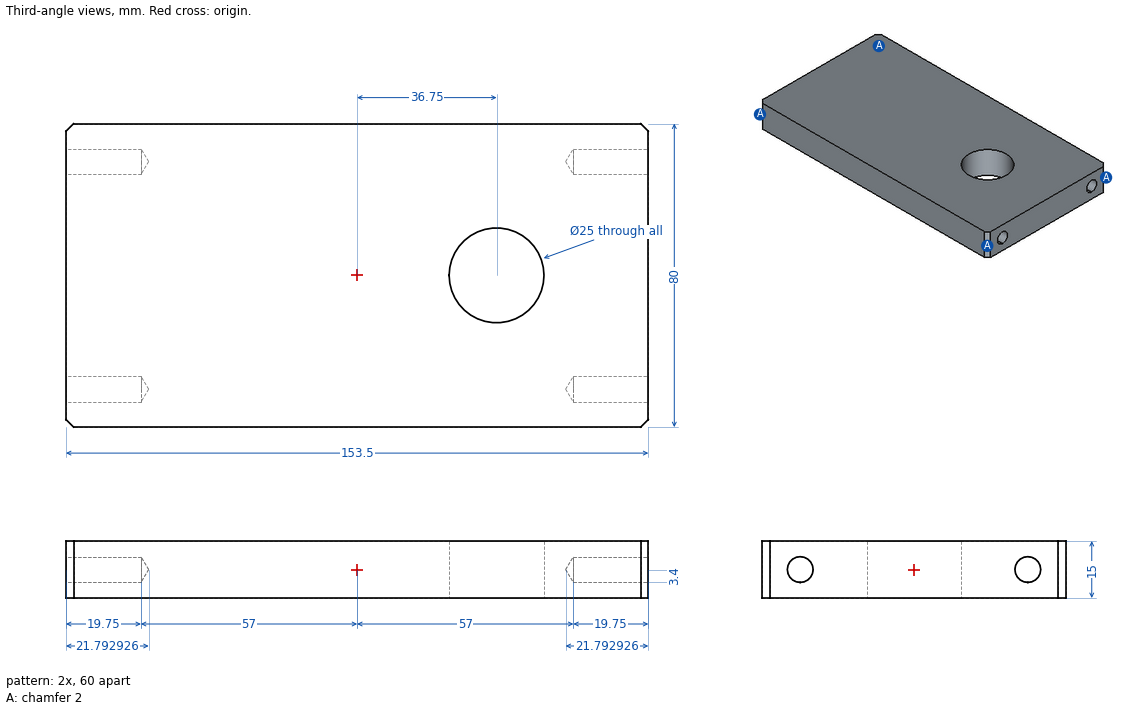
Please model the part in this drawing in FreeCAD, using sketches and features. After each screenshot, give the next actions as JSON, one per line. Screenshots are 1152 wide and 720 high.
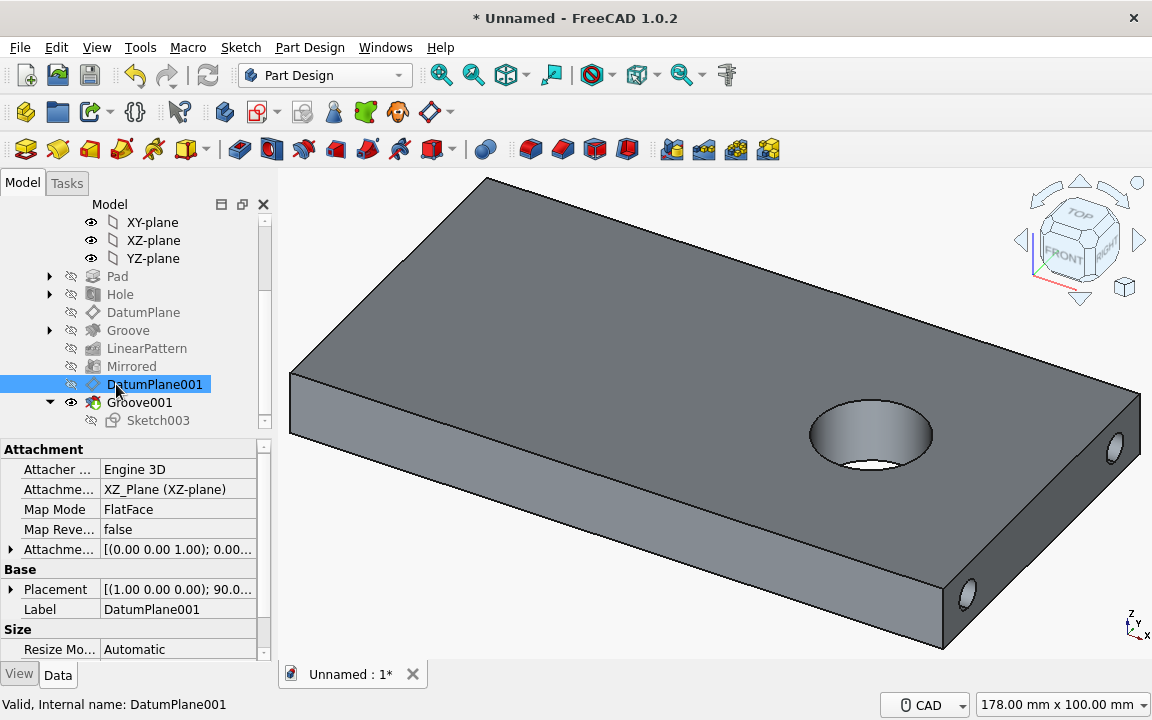
{"action": "left_click", "coordinate": [943, 618]}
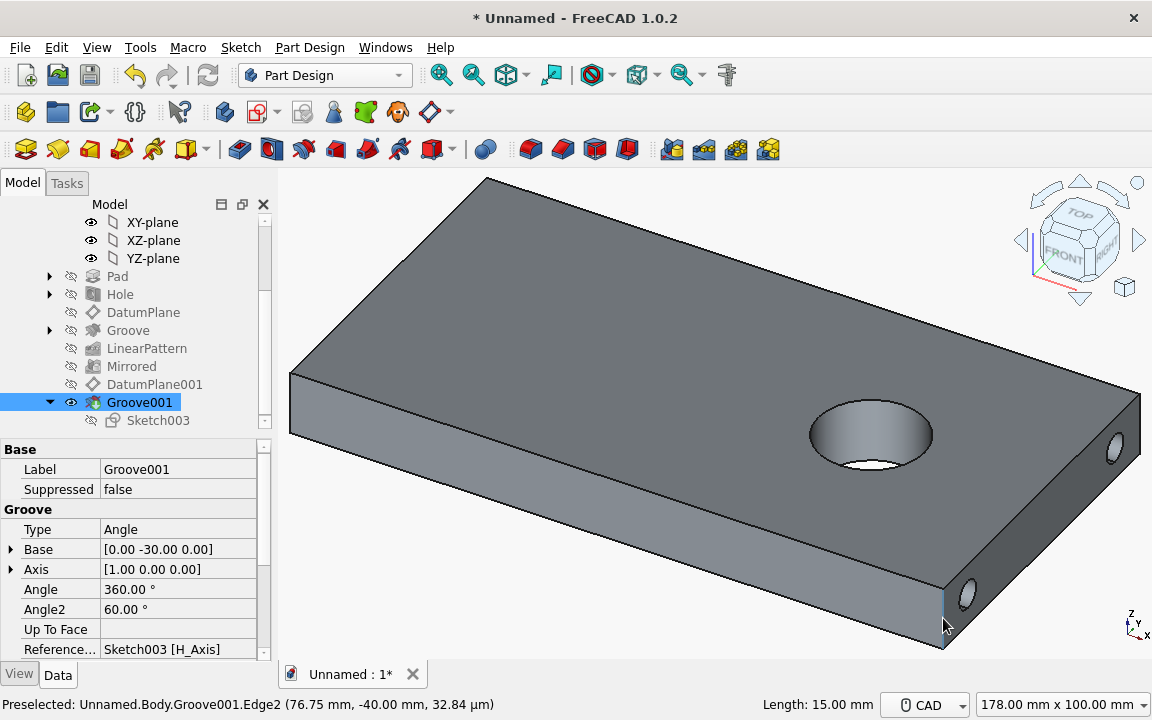
{"action": "key", "text": "0"}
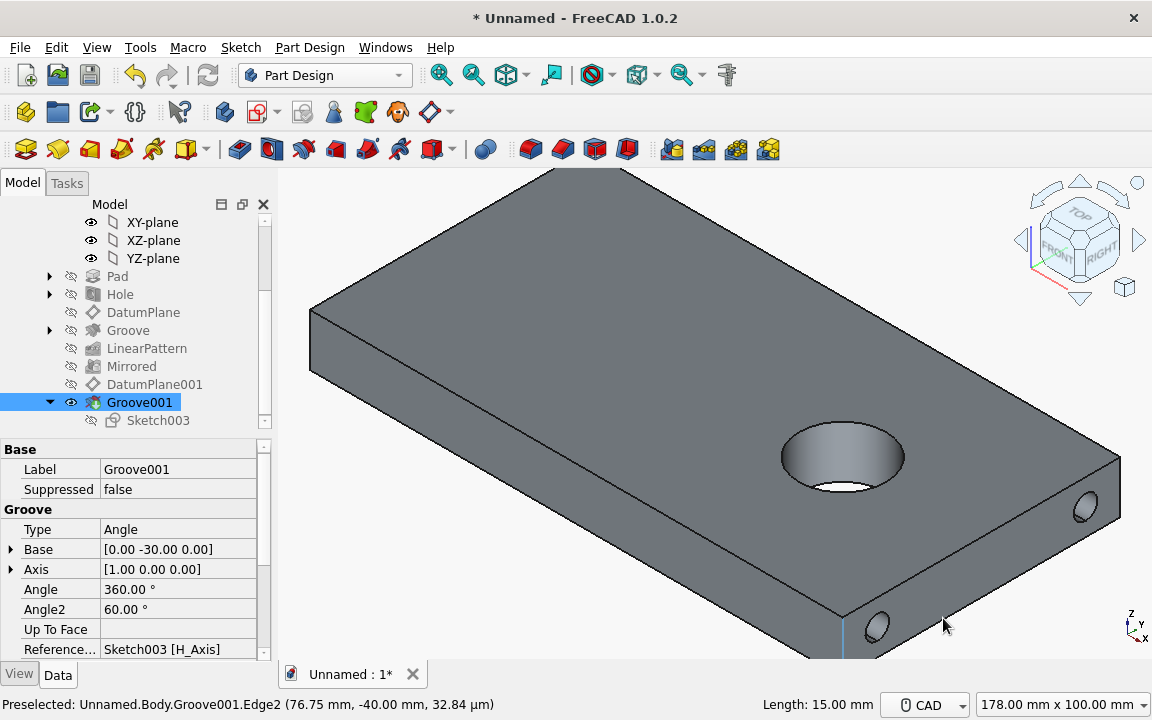
{"action": "left_click", "coordinate": [442, 76]}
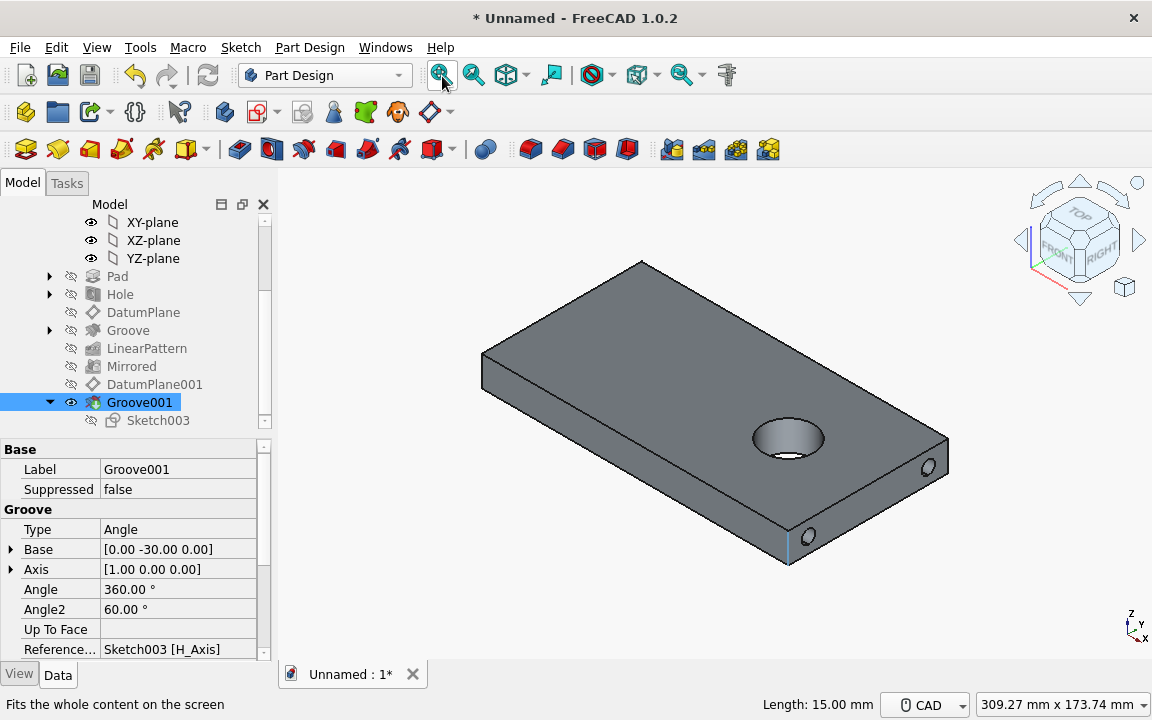
{"action": "key", "text": "2"}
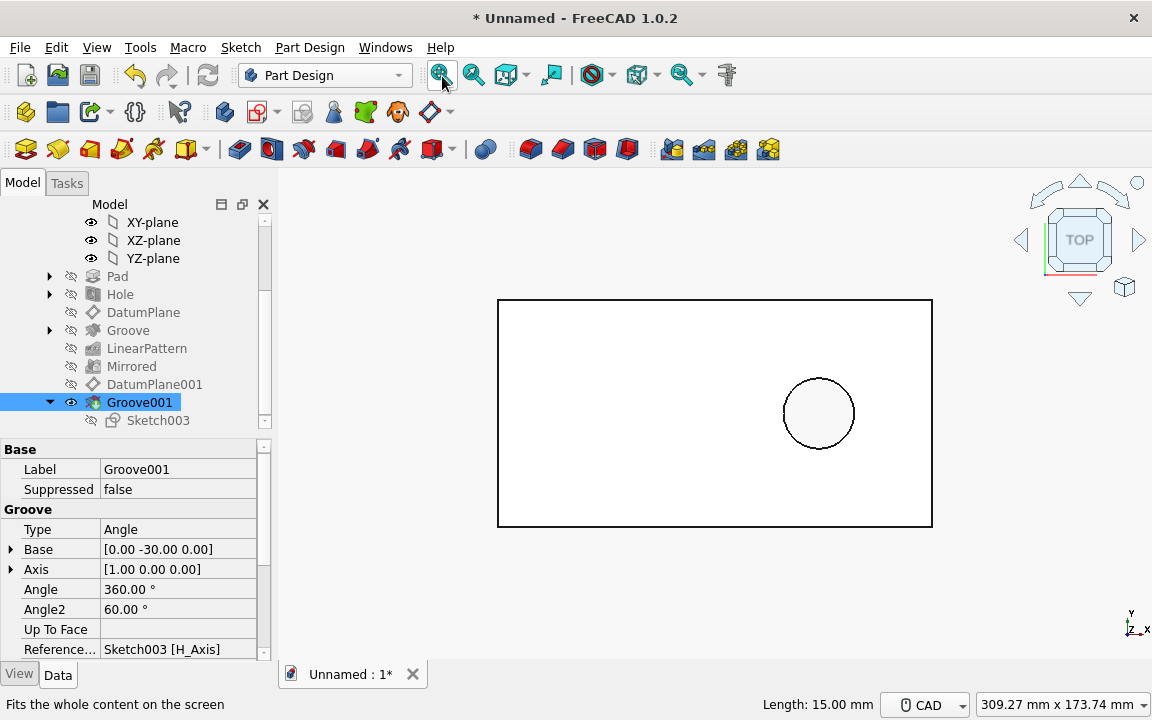
{"action": "key", "text": "1"}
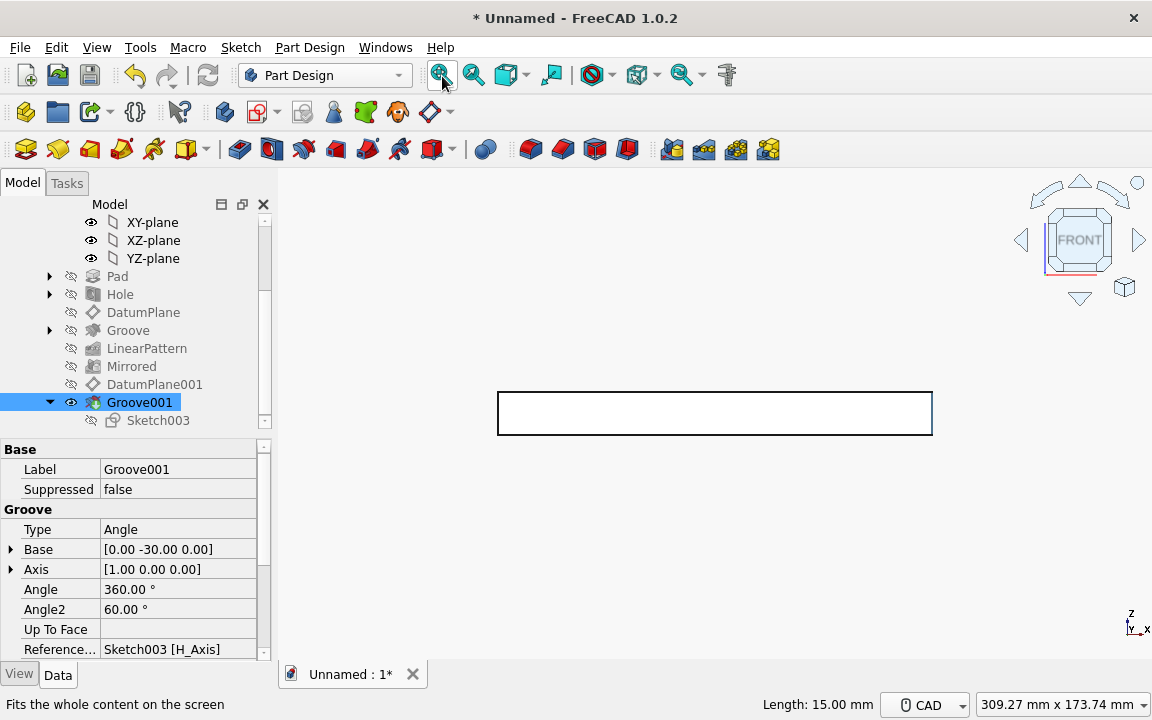
{"action": "left_click", "coordinate": [498, 413], "text": "ctrl"}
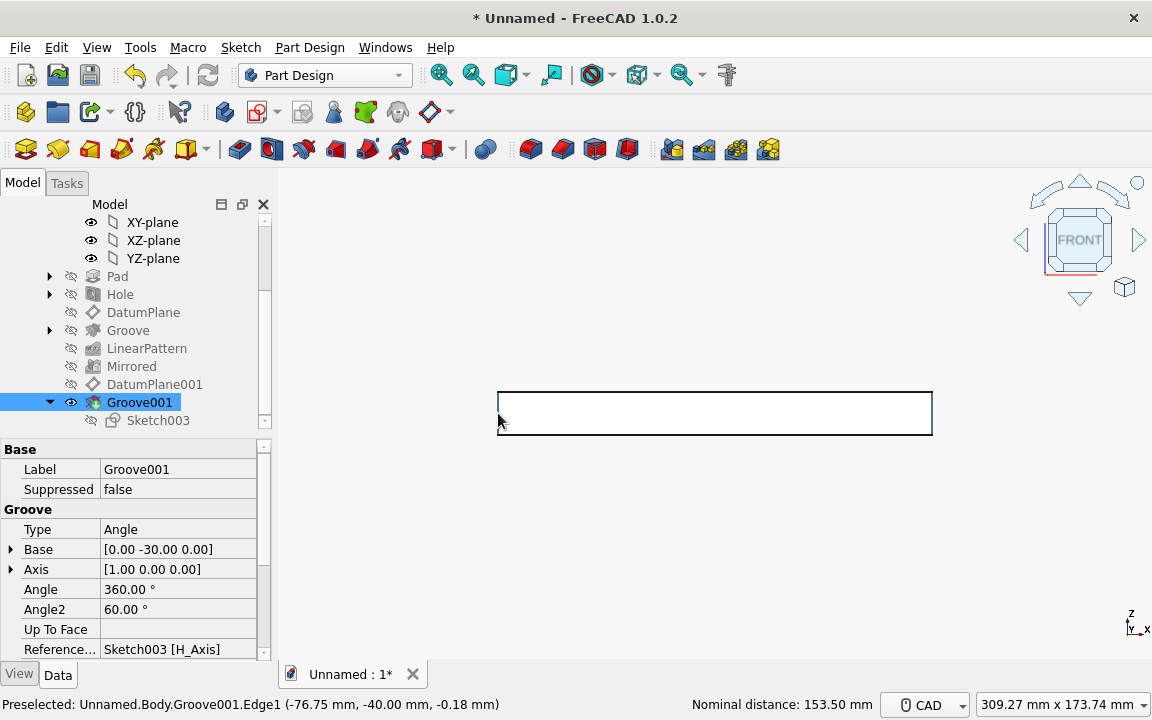
{"action": "key", "text": "3"}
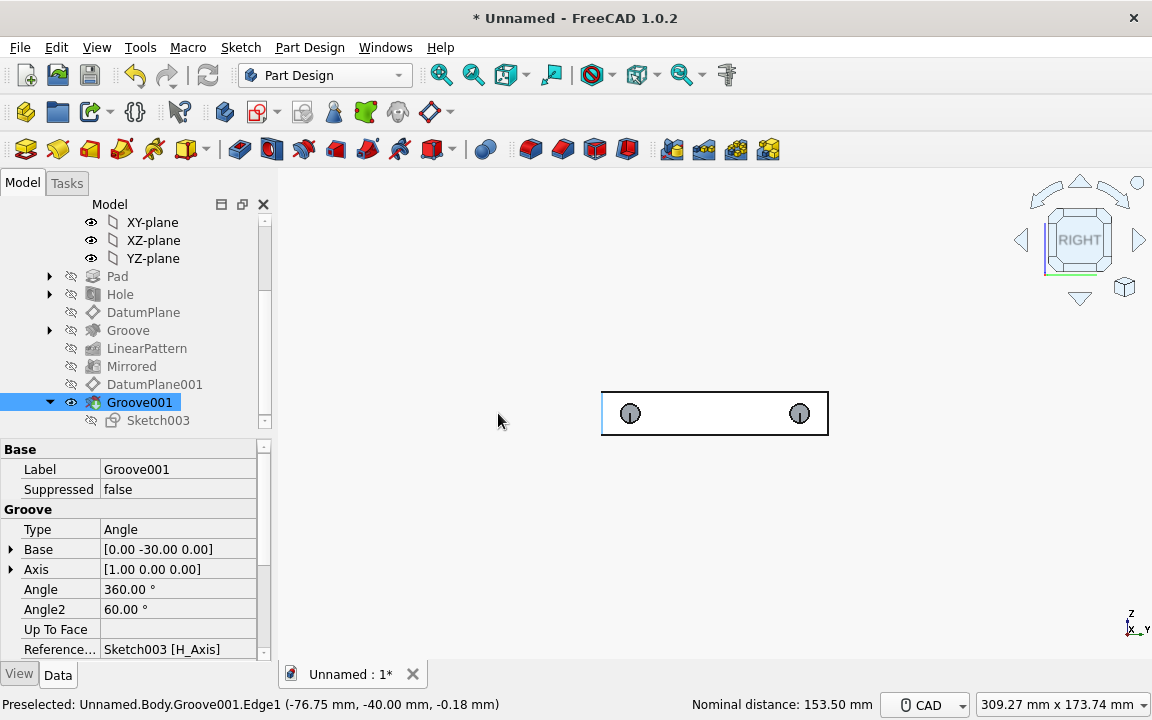
{"action": "key", "text": "v f"}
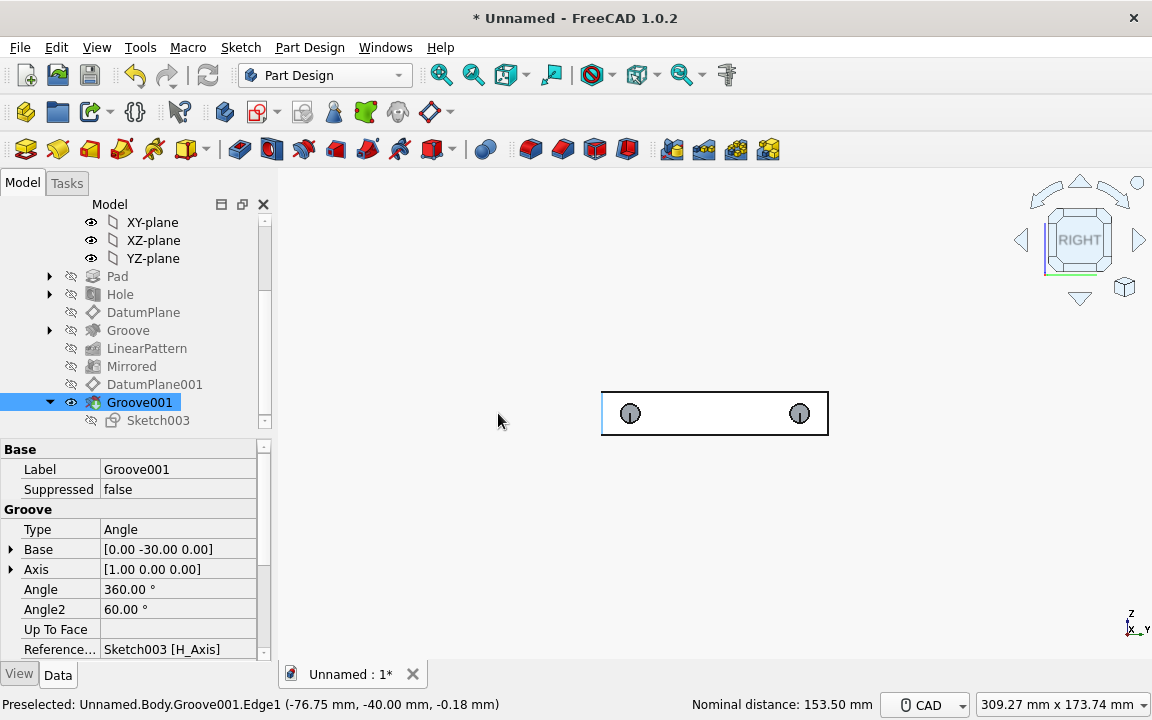
{"action": "left_click", "coordinate": [828, 412], "text": "ctrl"}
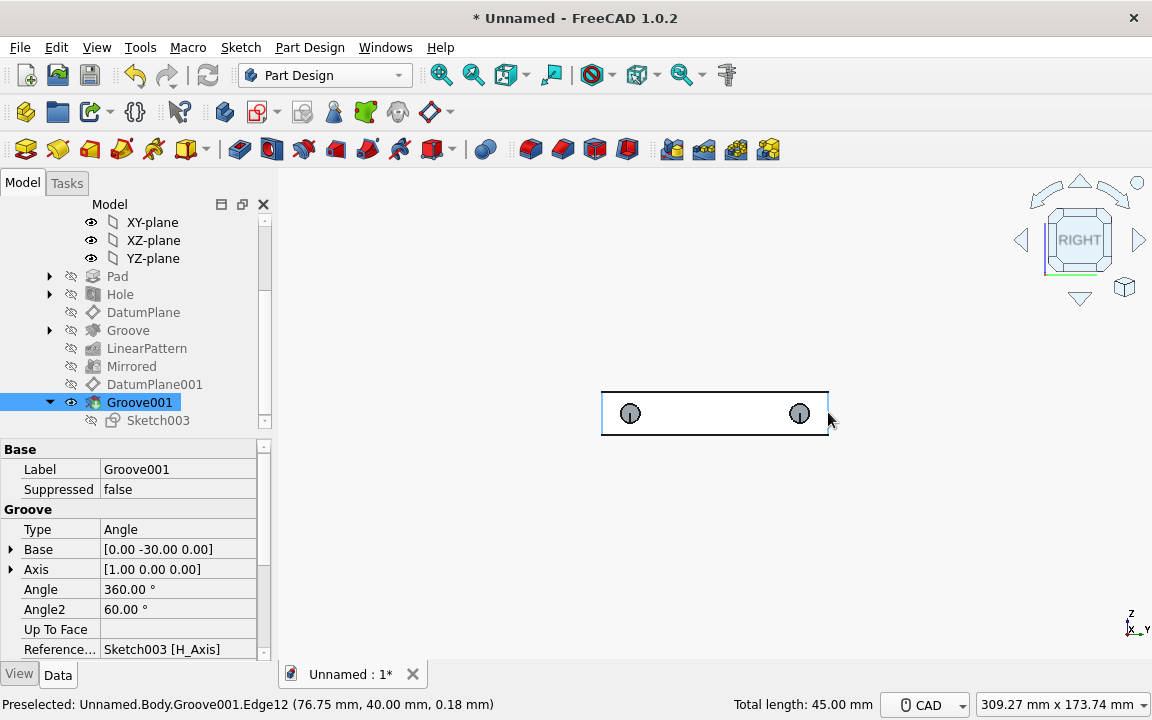
{"action": "key", "text": "5"}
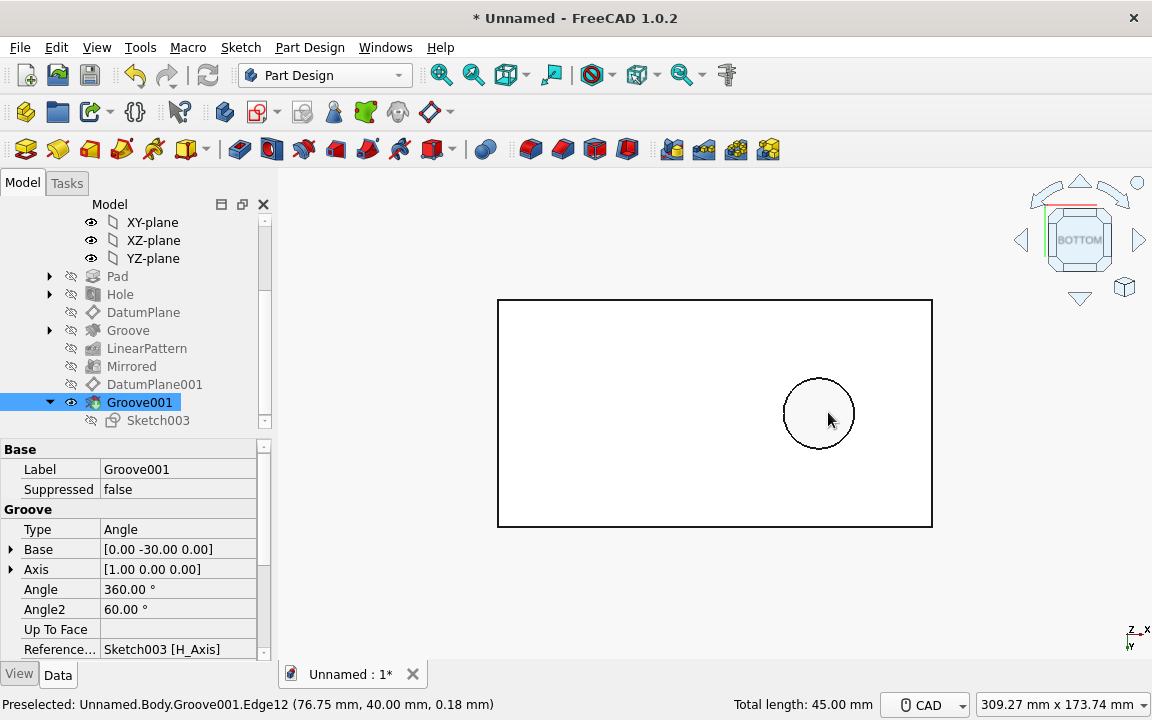
{"action": "key", "text": "4"}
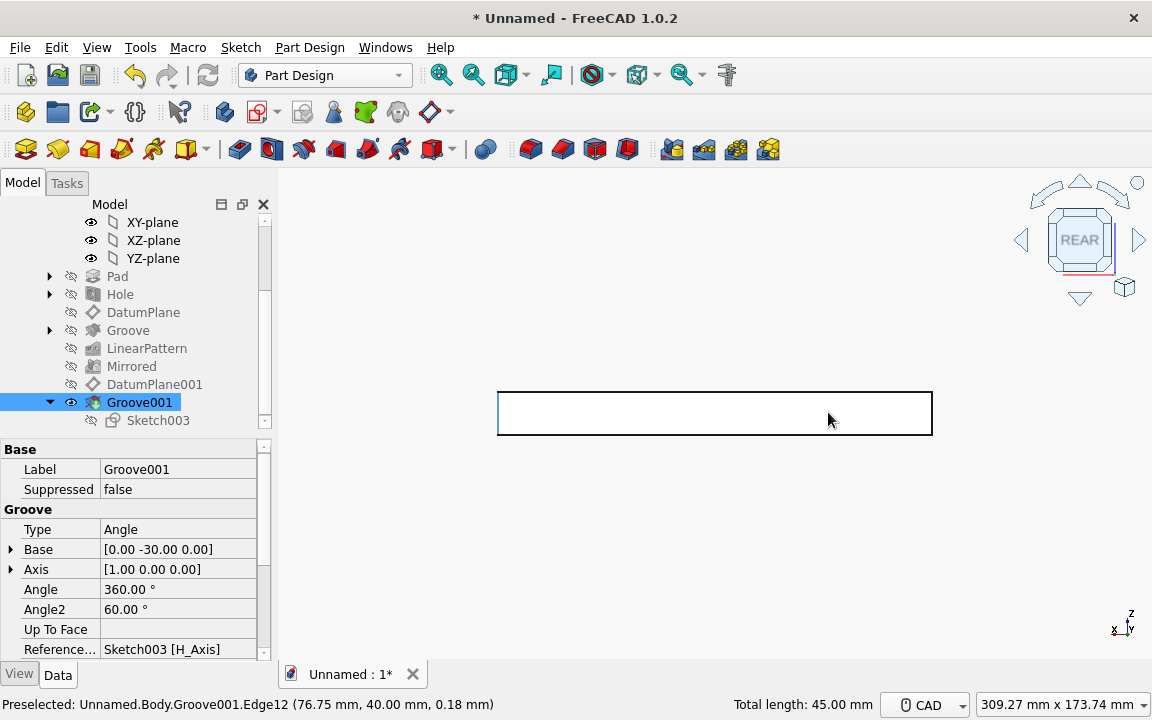
{"action": "left_click", "coordinate": [932, 413], "text": "ctrl"}